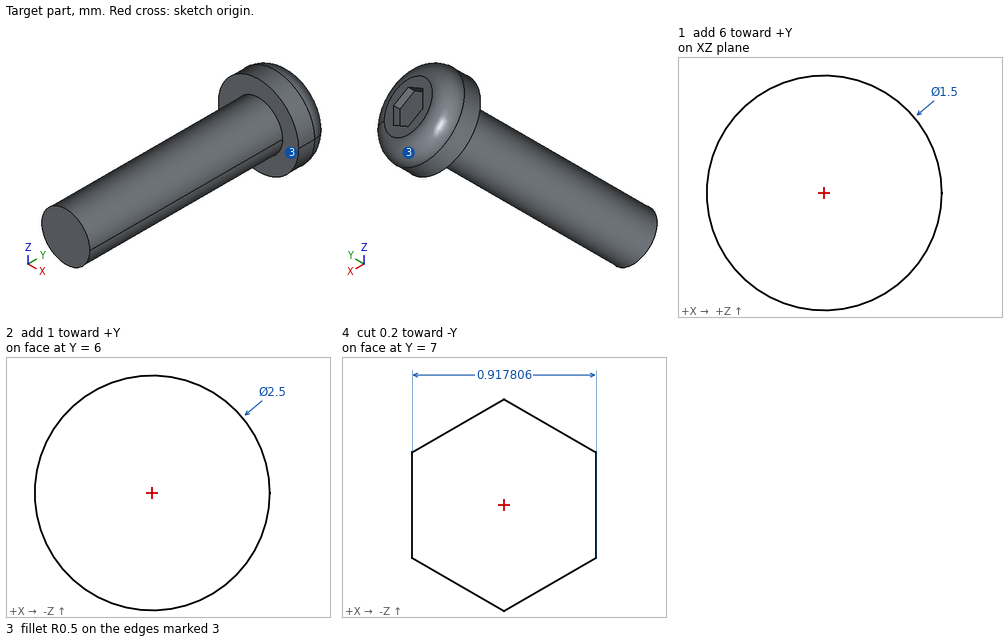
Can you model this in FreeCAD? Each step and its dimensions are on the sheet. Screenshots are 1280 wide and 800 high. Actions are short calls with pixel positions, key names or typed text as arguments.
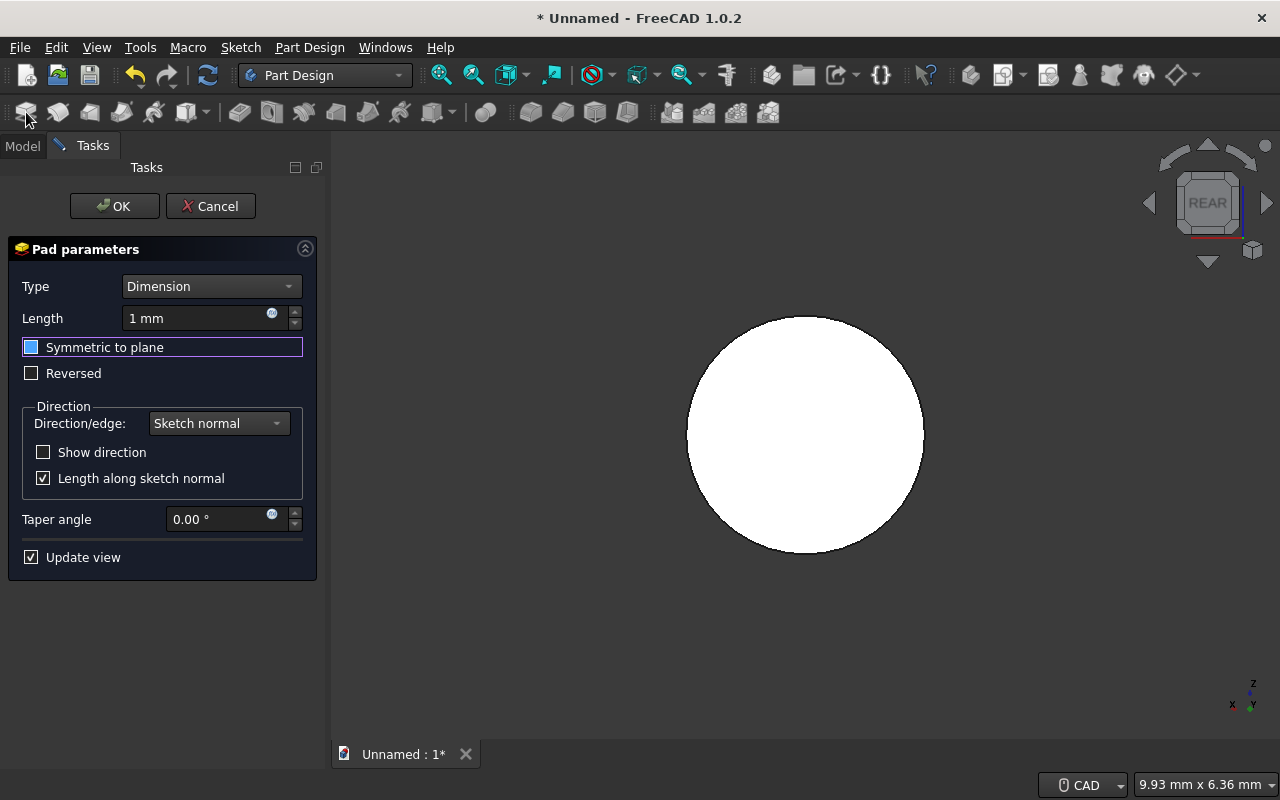
click(115, 206)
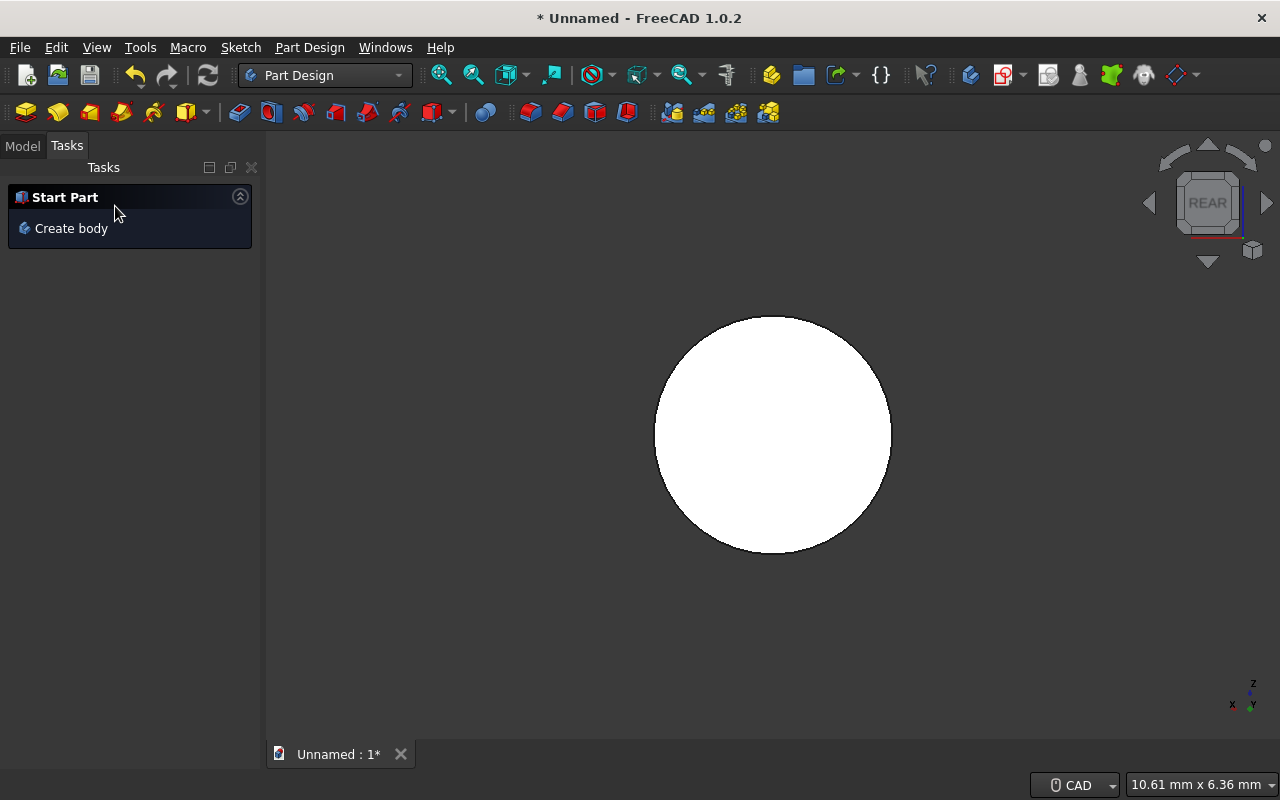
key(v)
key(f)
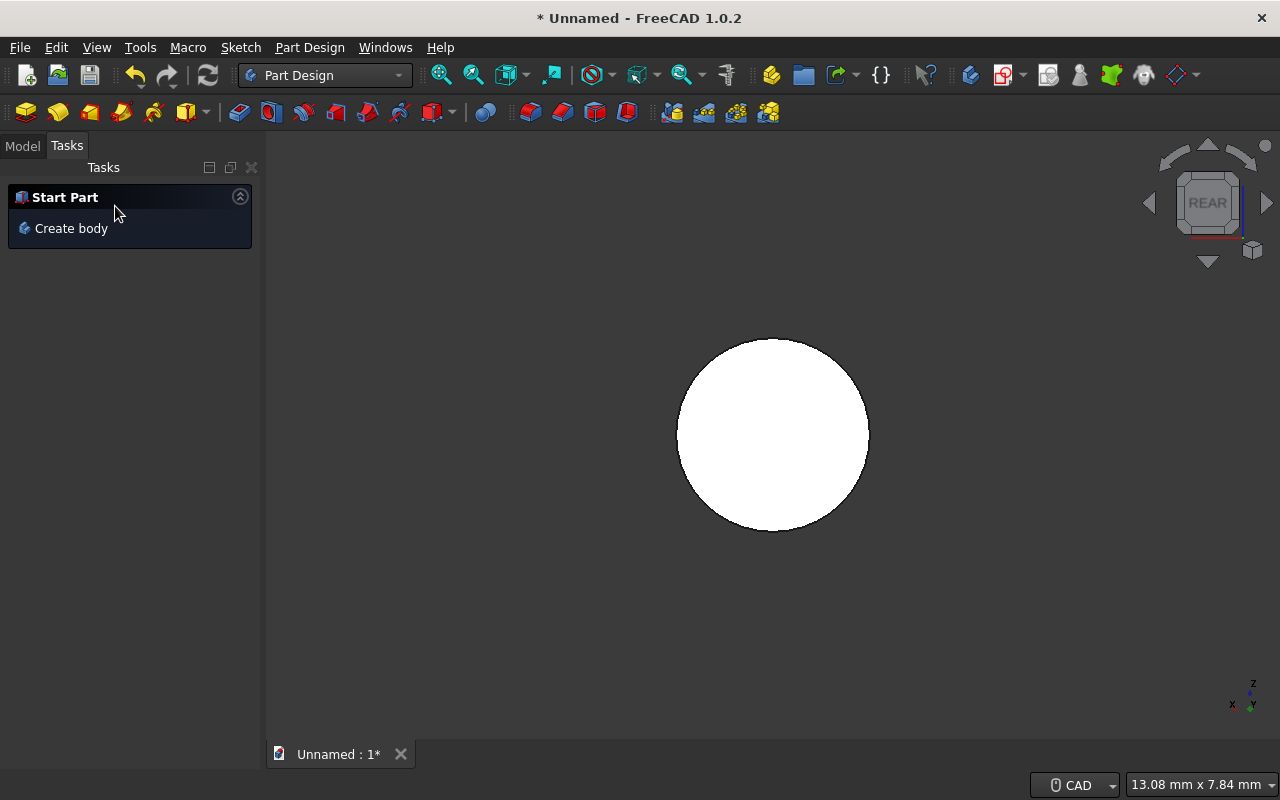
click(870, 434)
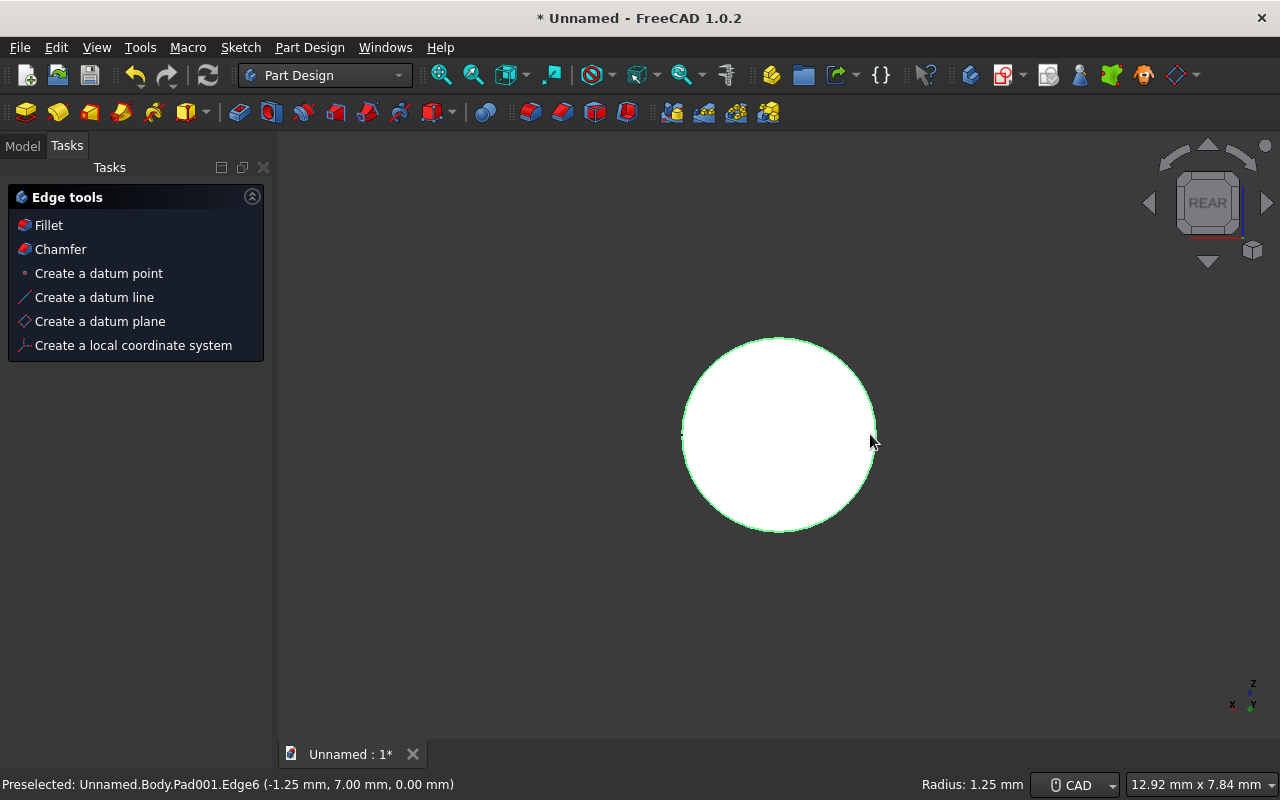
click(532, 112)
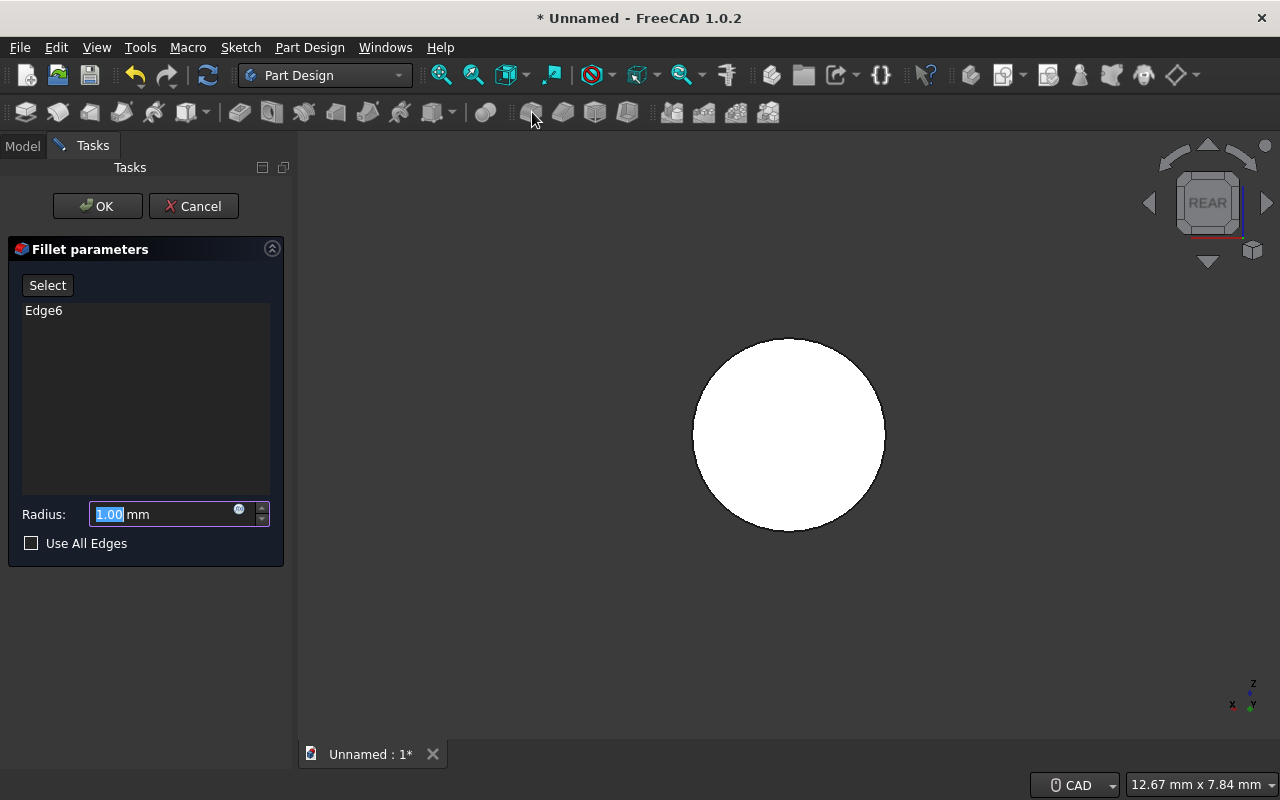
text(0.5)
key(Tab)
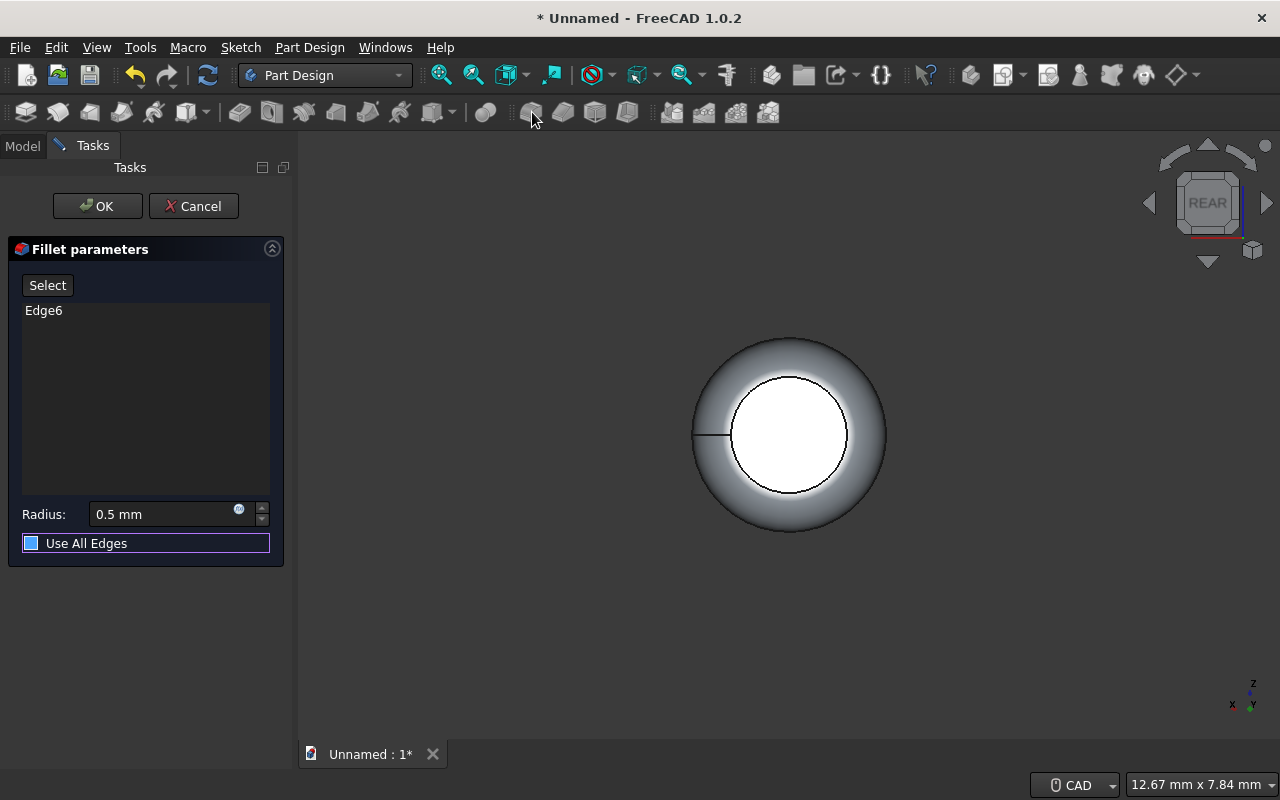
click(98, 206)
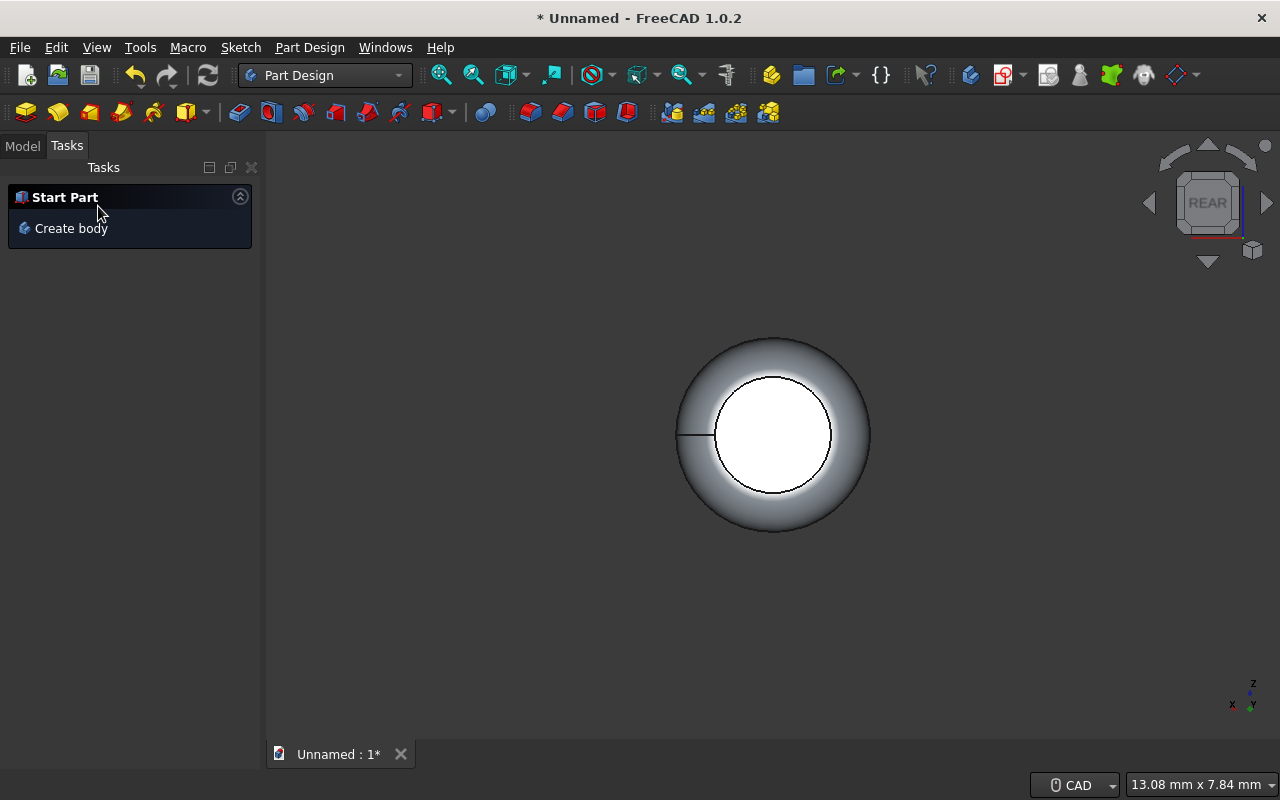
click(442, 76)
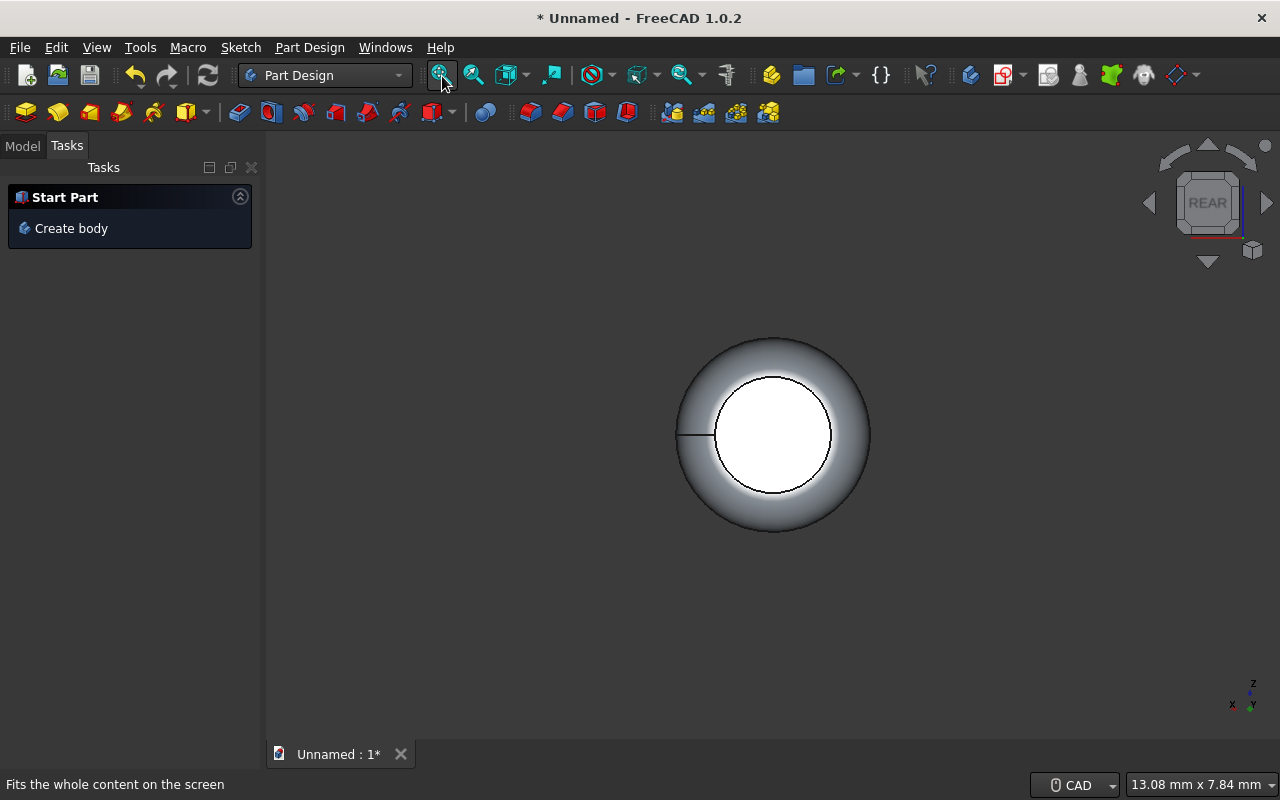
click(773, 434)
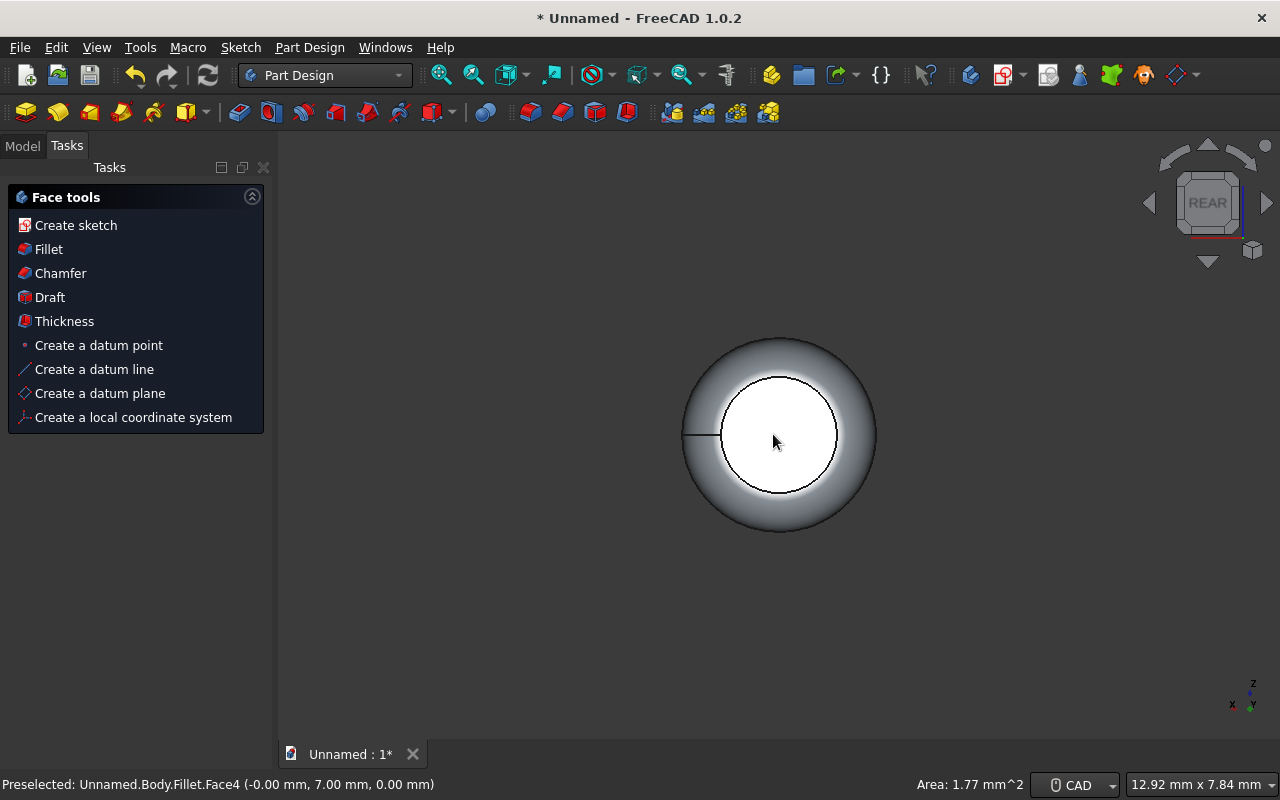
click(1004, 76)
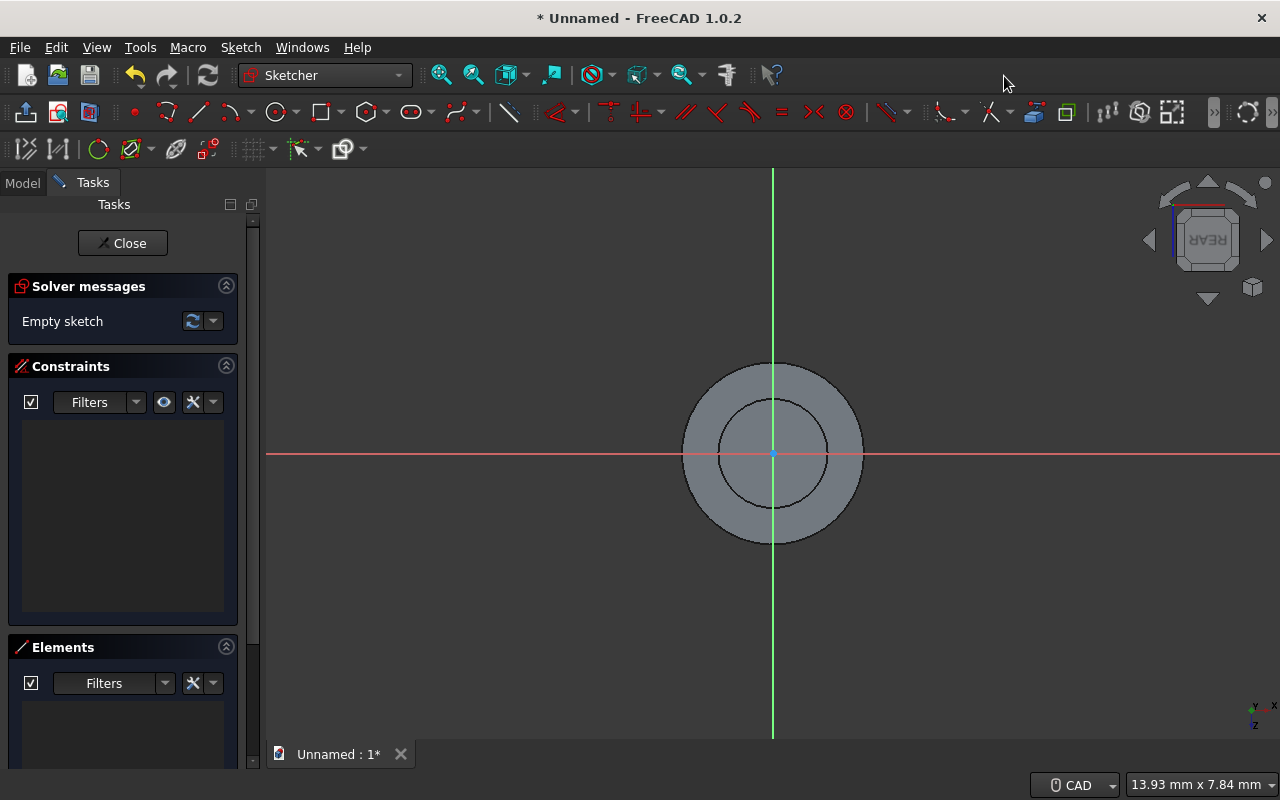
scroll(790, 453, up, 8)